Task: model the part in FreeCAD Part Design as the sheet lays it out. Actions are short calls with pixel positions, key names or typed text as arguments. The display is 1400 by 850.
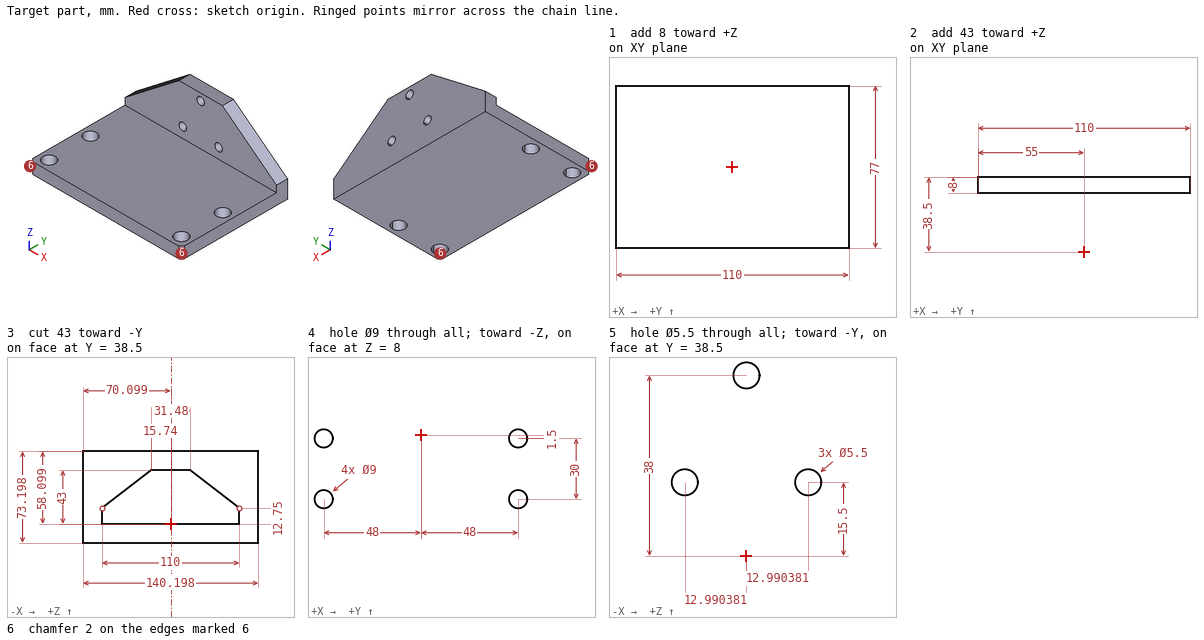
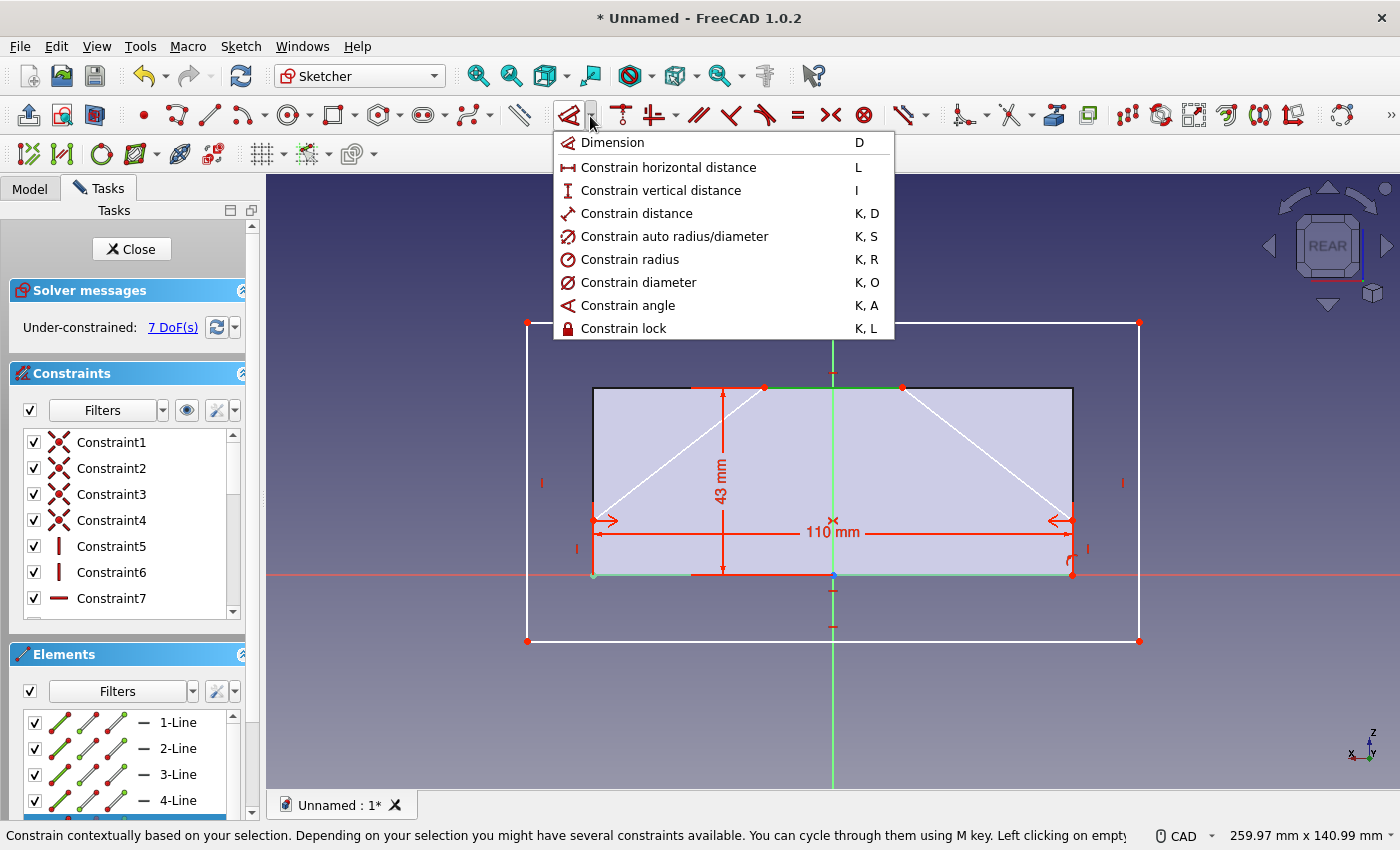
click(724, 168)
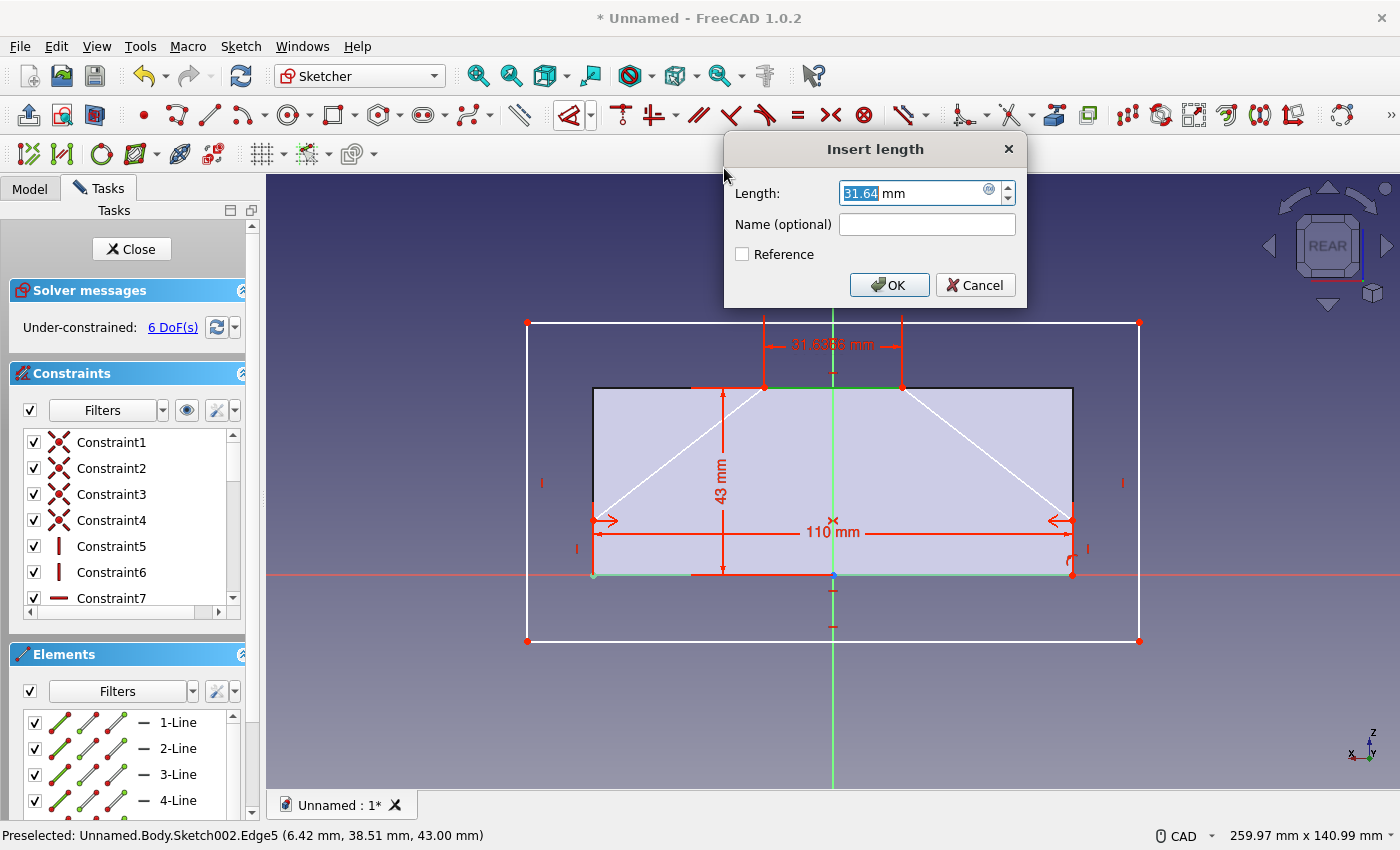
text(31.48)
key(Return)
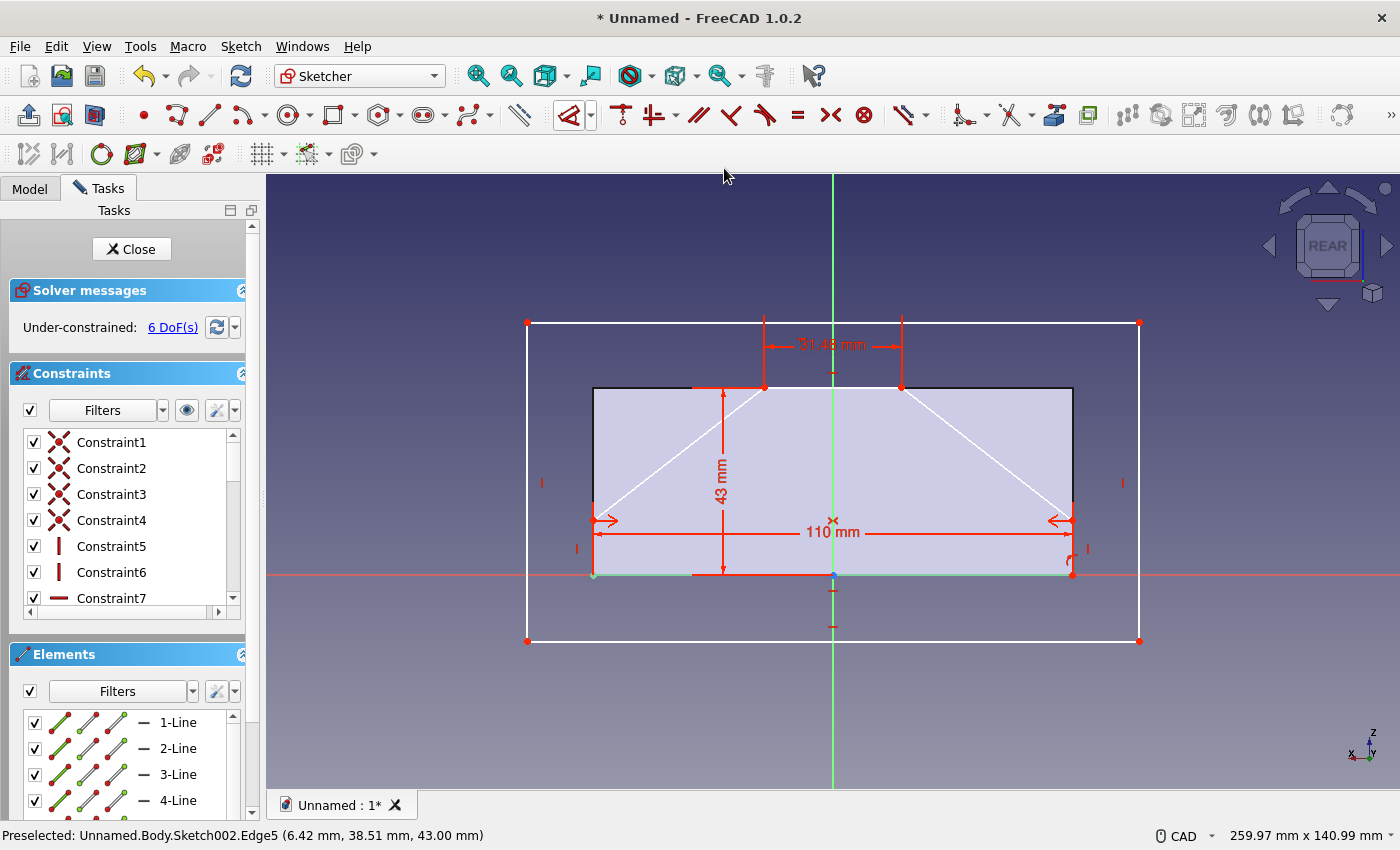
click(1073, 537)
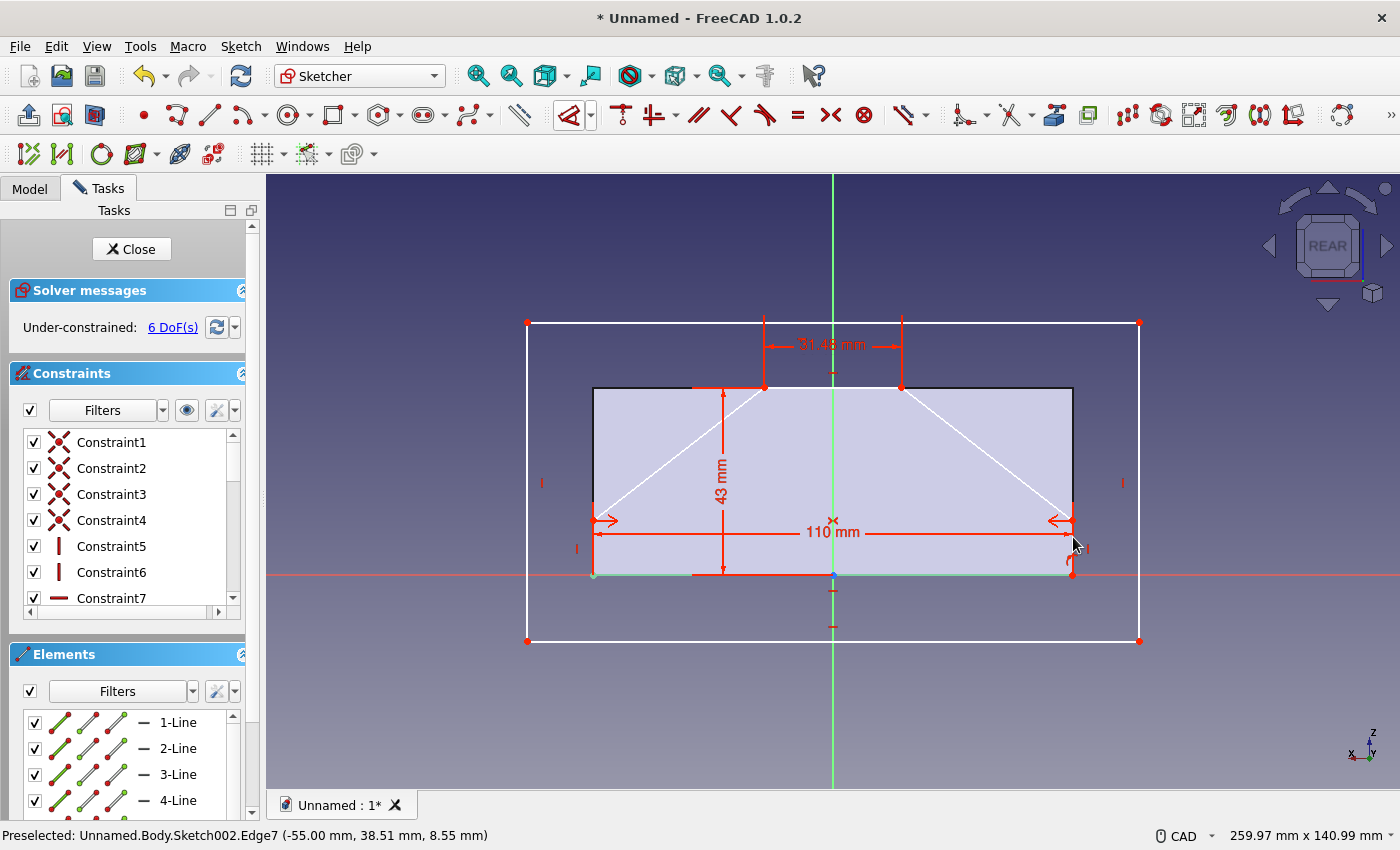
key(i)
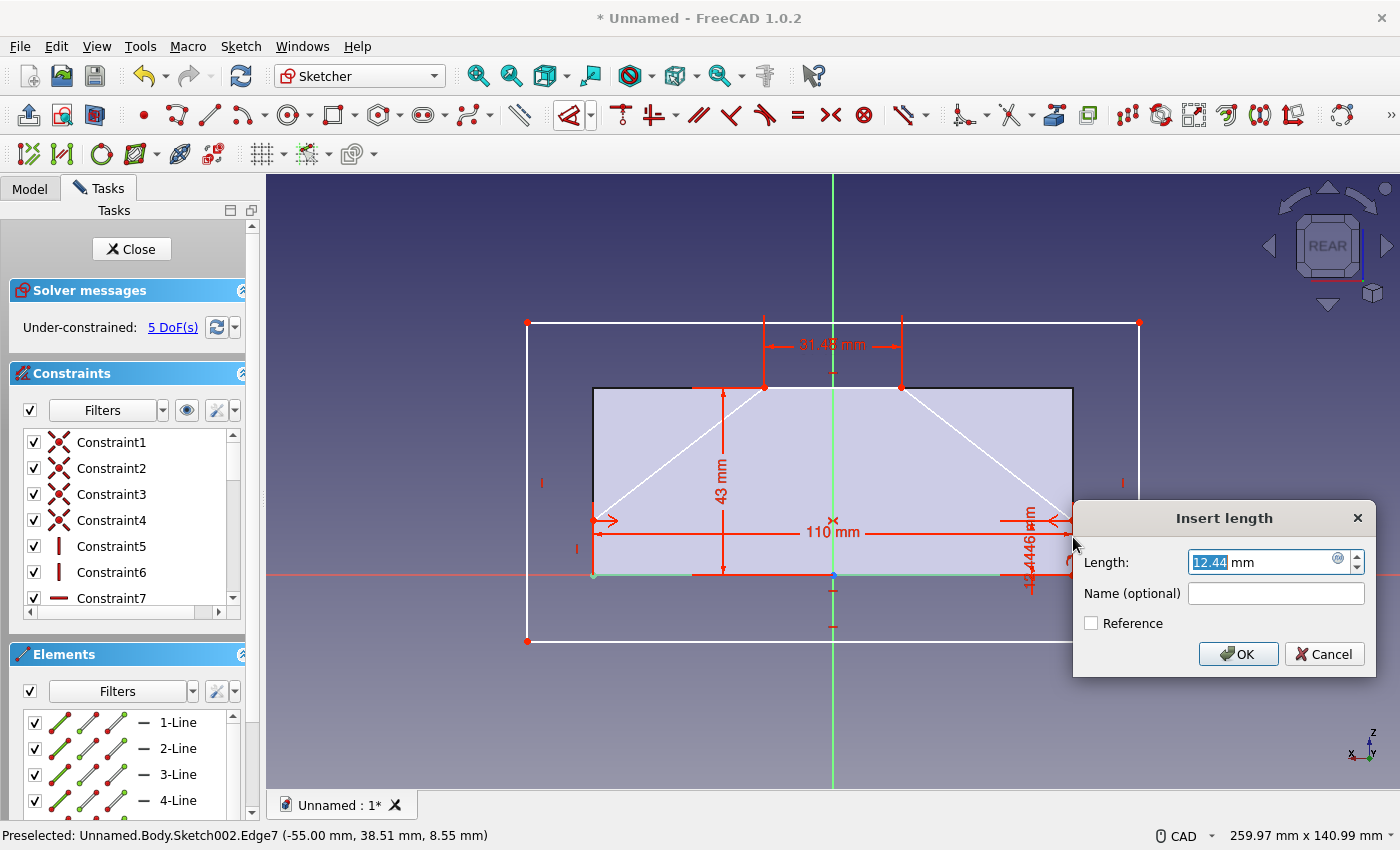
text(12.75)
key(Return)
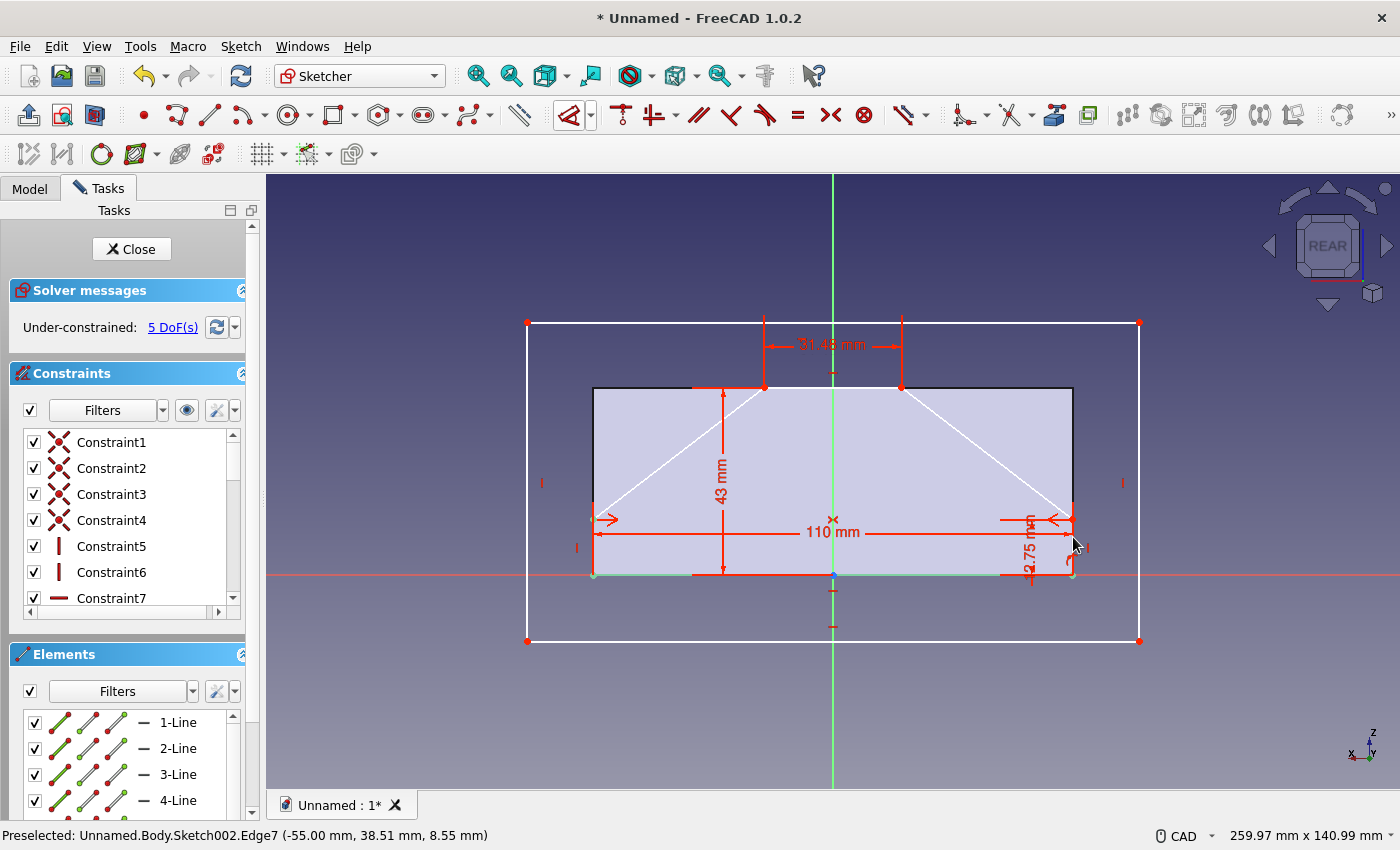
click(527, 419)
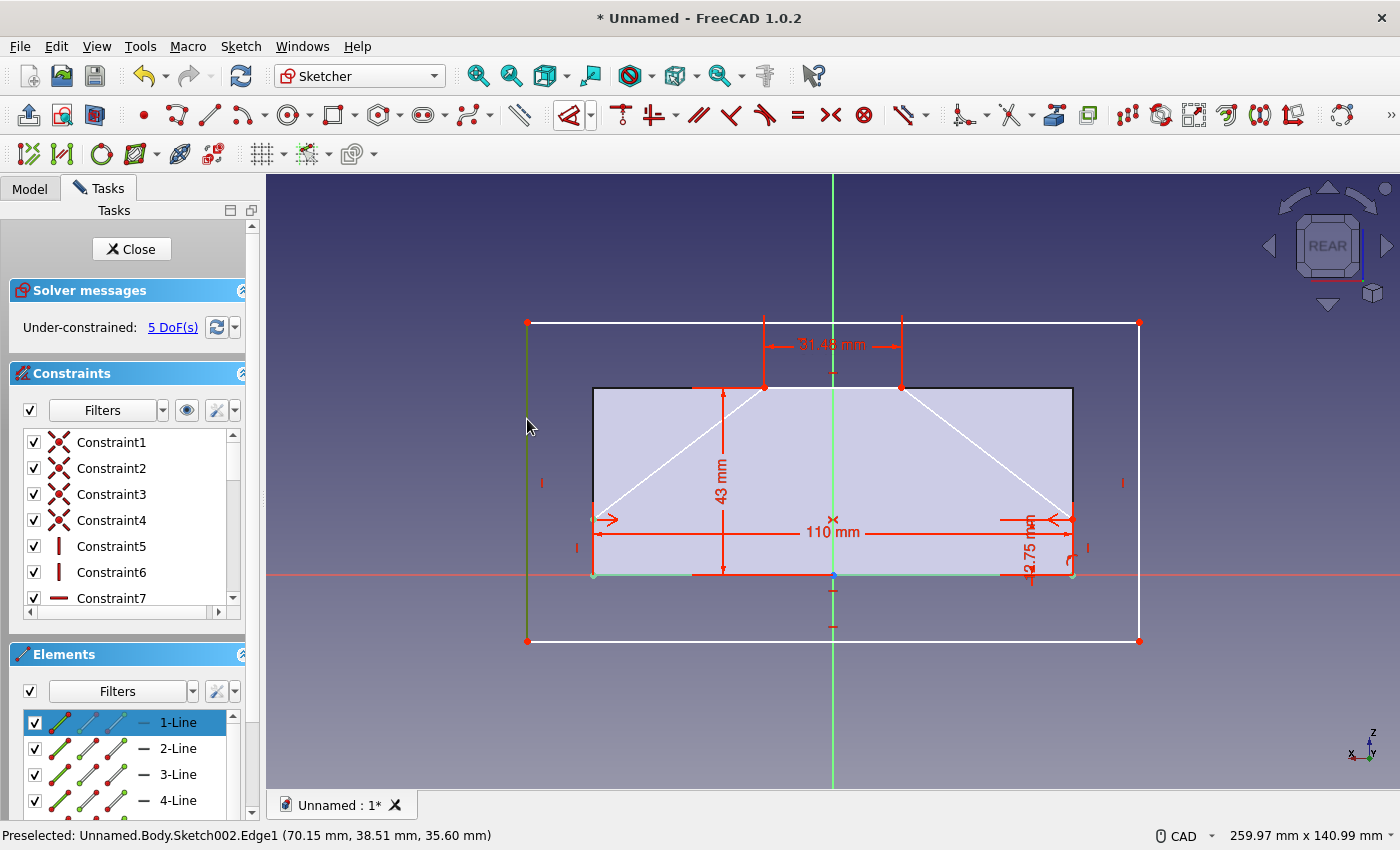
key(i)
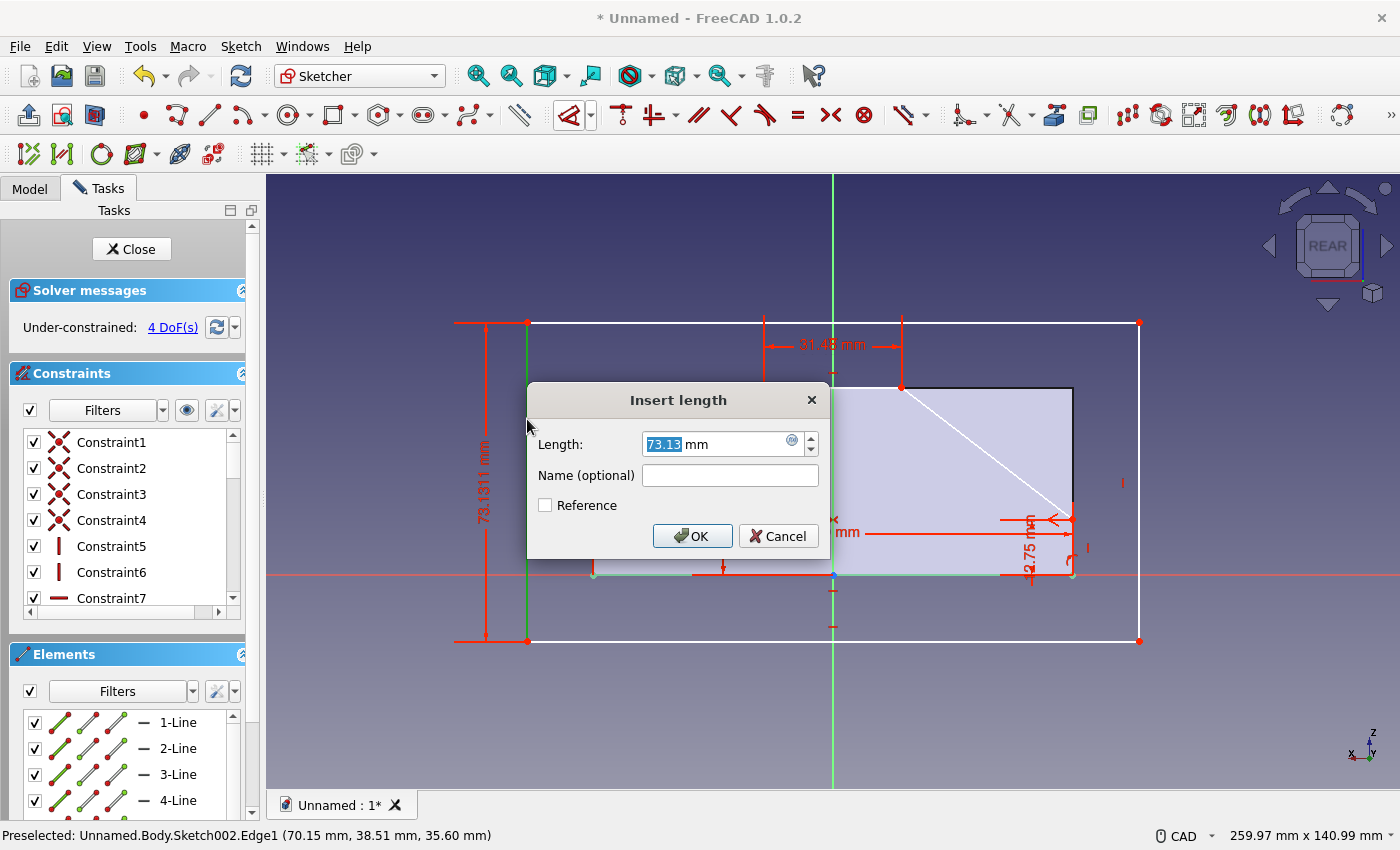
text(73.198)
key(Return)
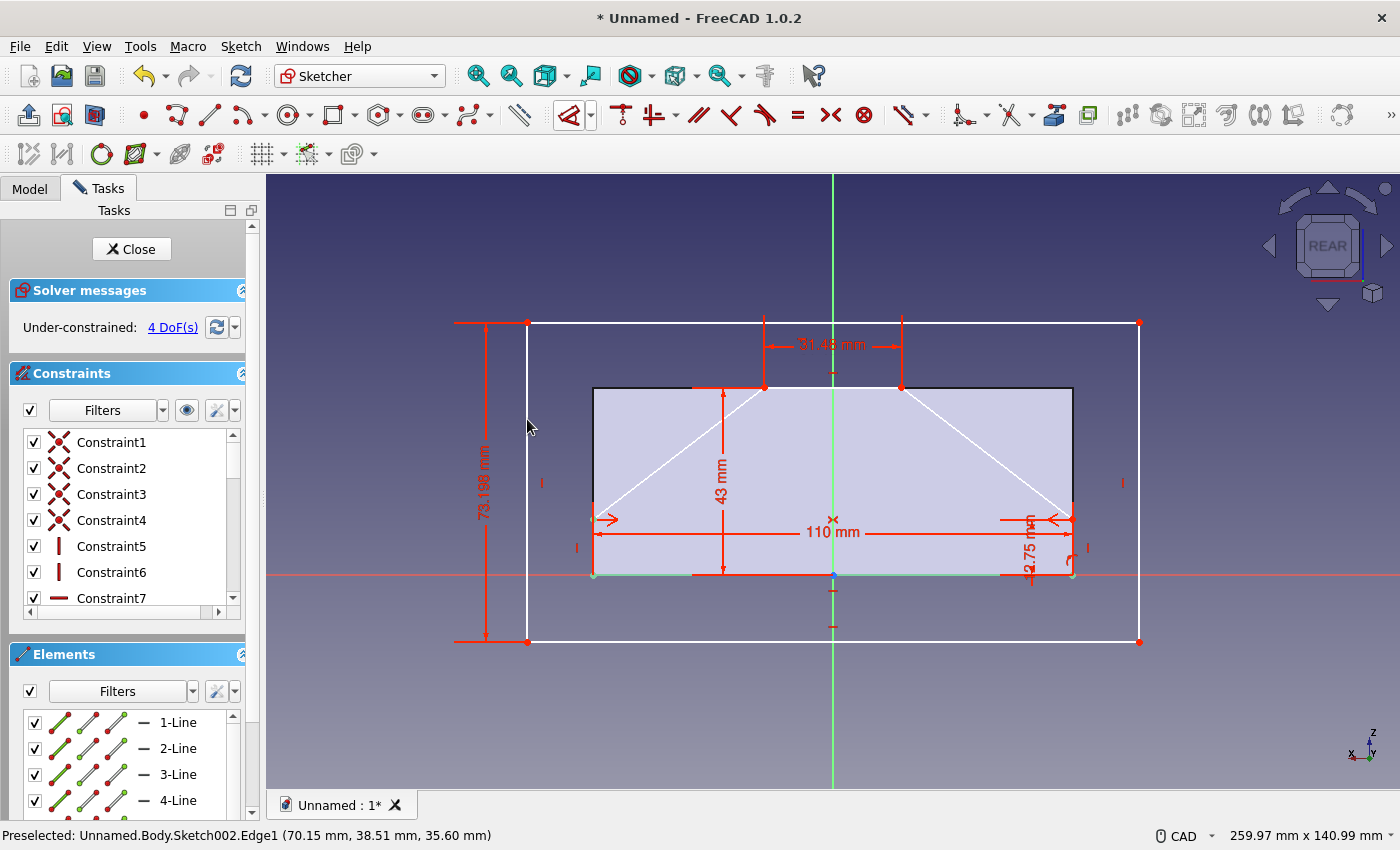
click(764, 388)